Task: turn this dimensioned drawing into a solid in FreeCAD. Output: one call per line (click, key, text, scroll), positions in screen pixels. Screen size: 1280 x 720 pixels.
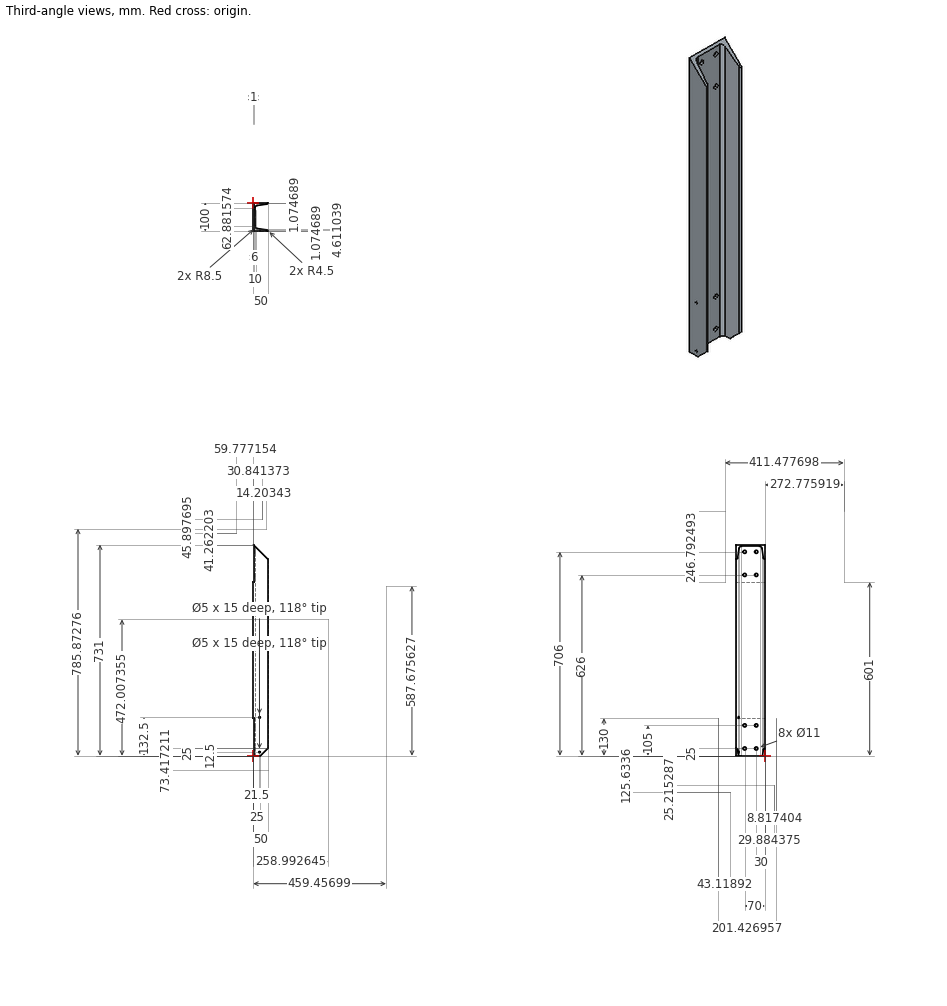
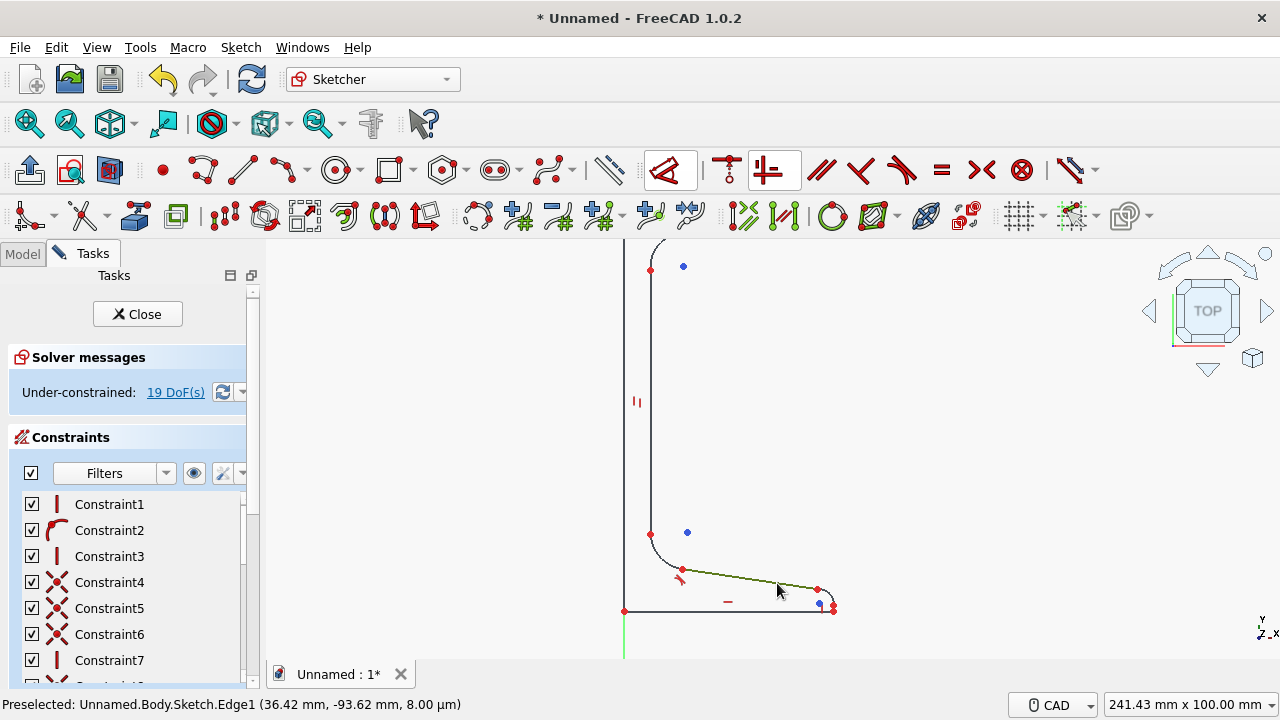
click(830, 594)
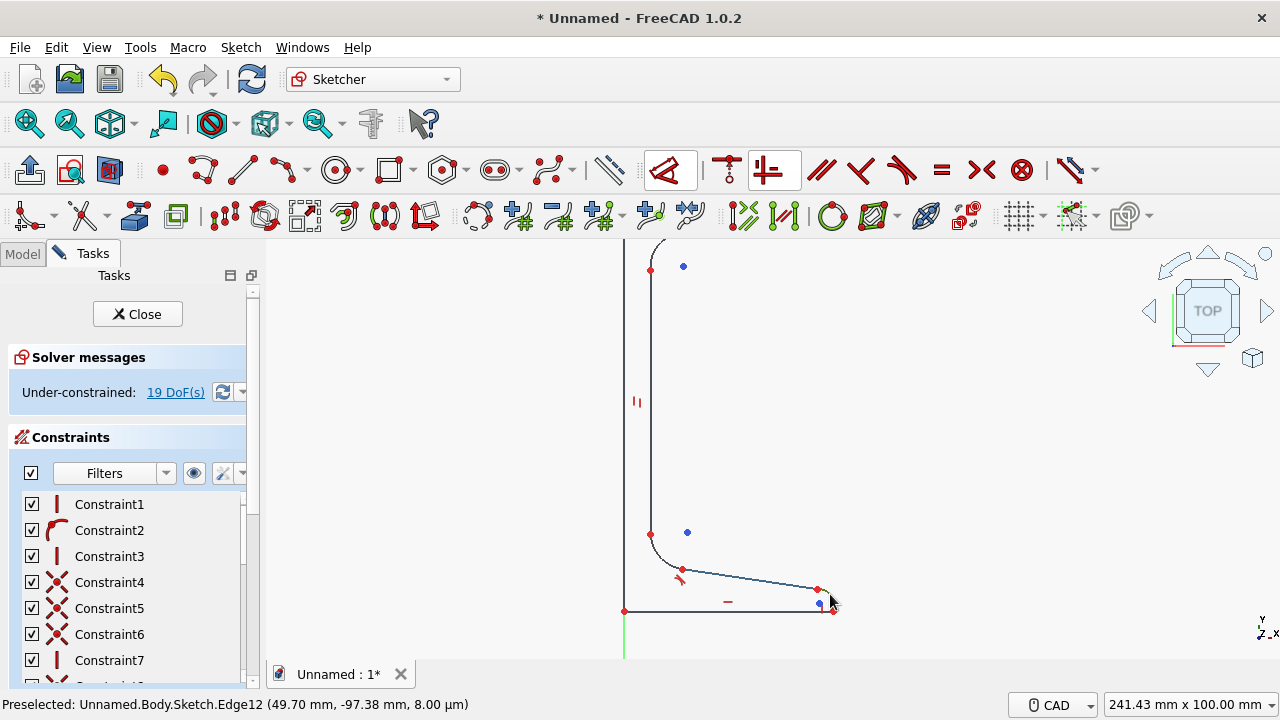
key(t)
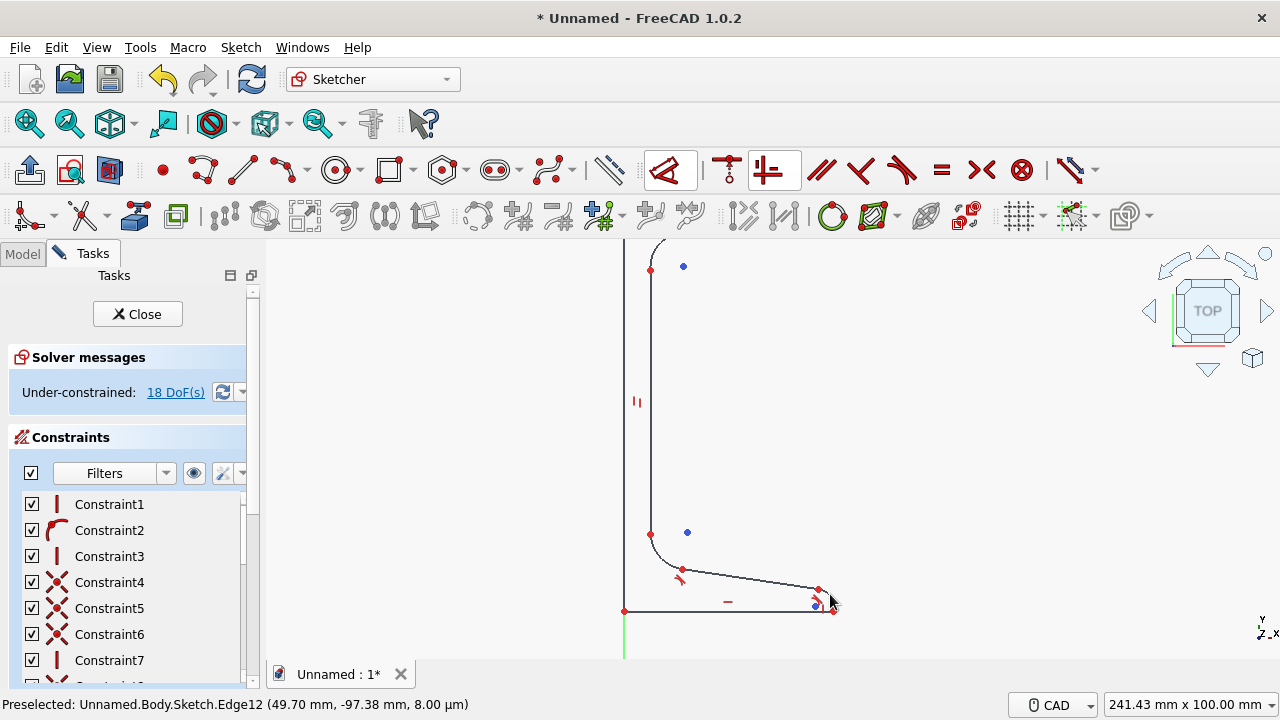
click(651, 455)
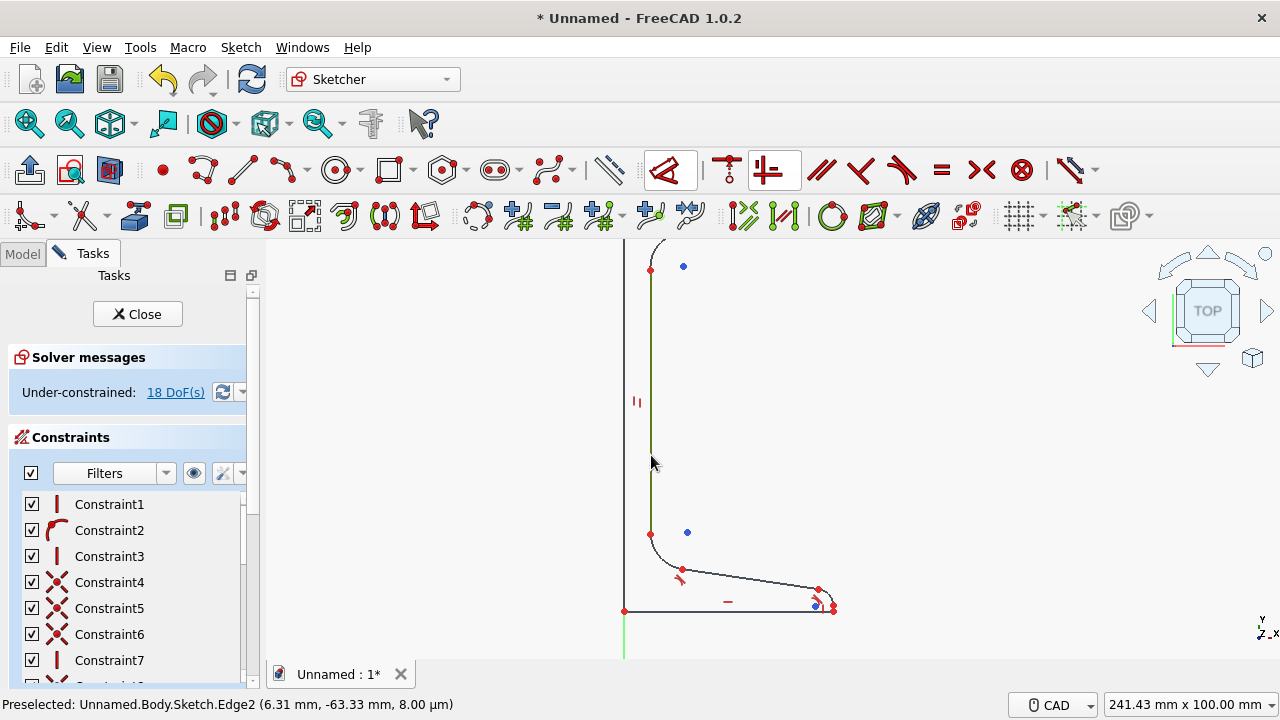
click(655, 549)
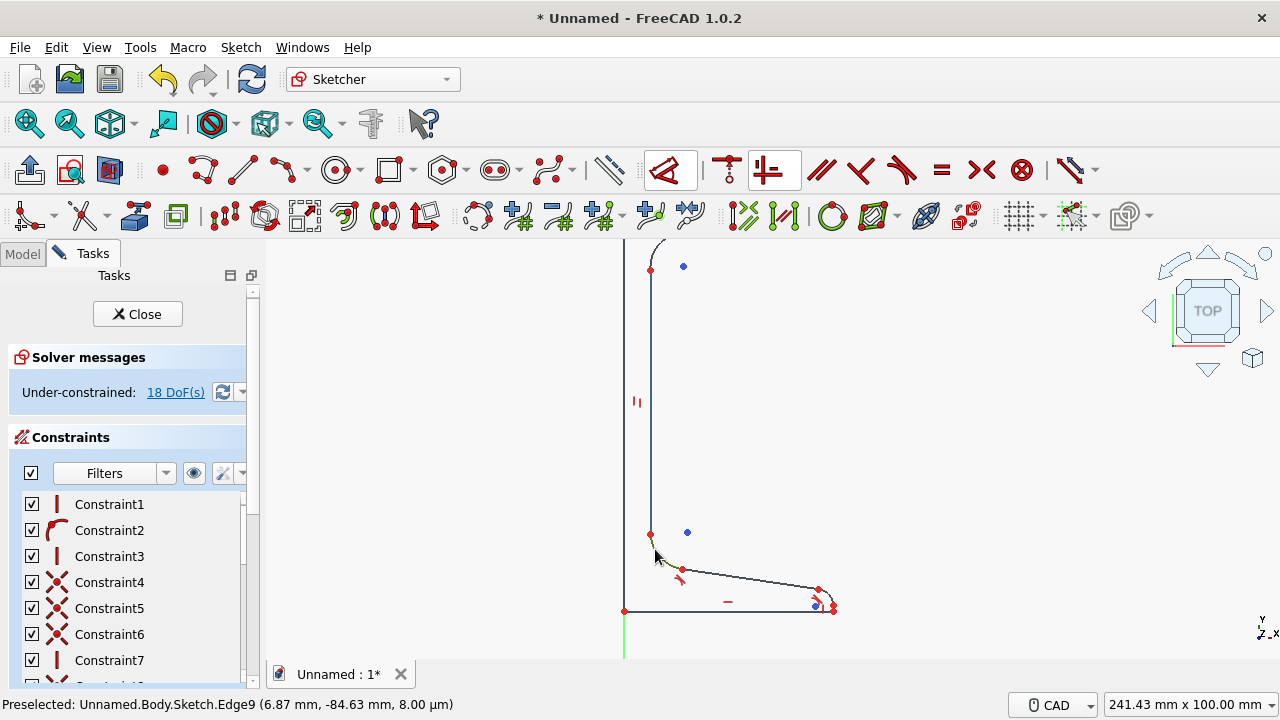
key(t)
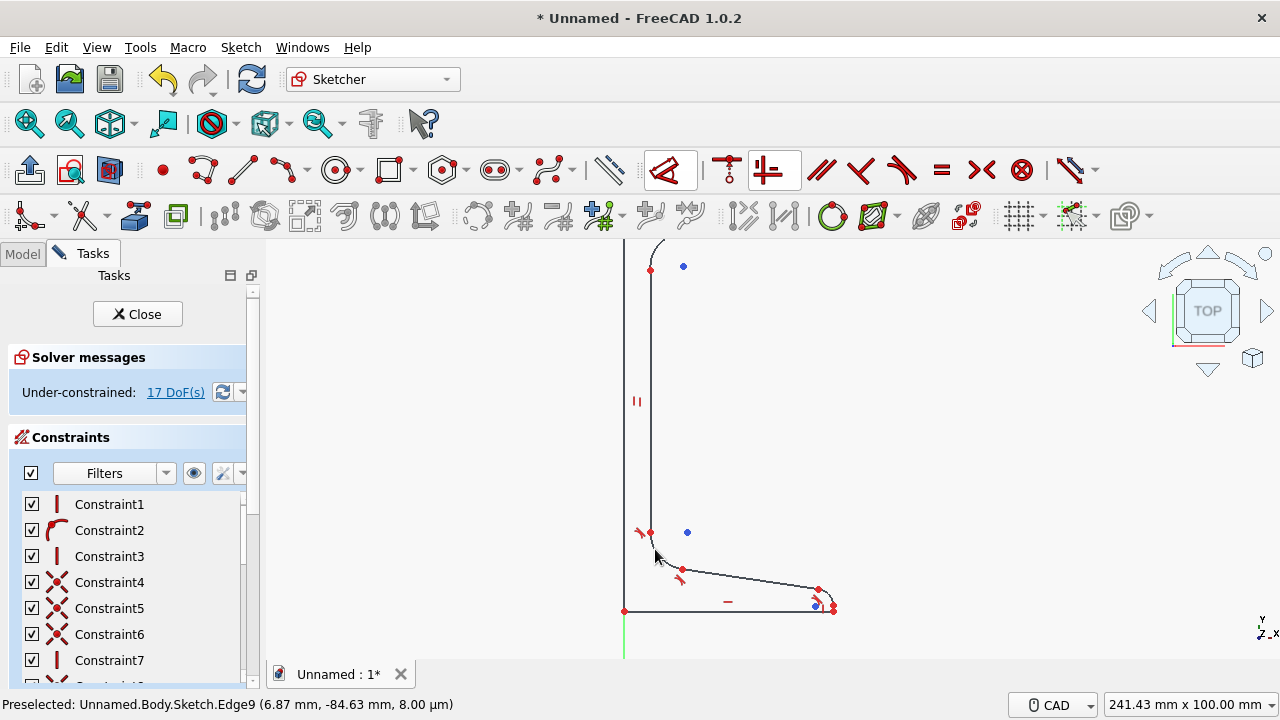
click(651, 454)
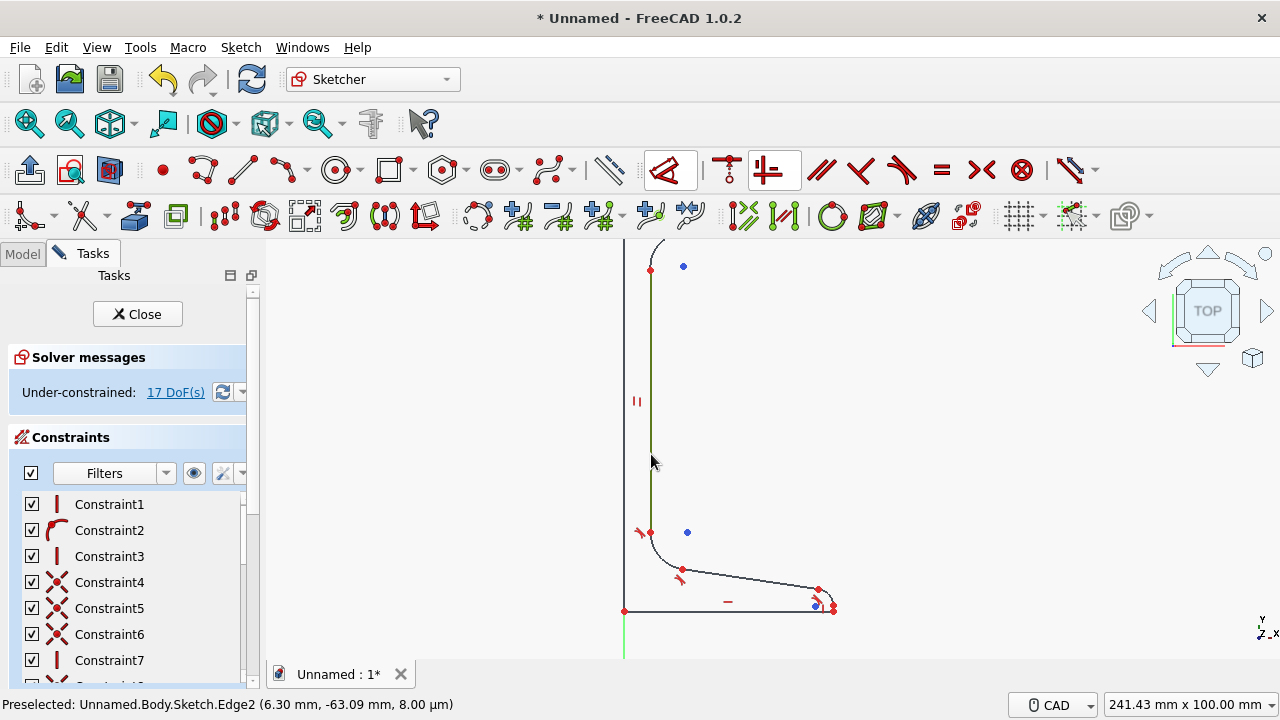
scroll(654, 549, down, 2)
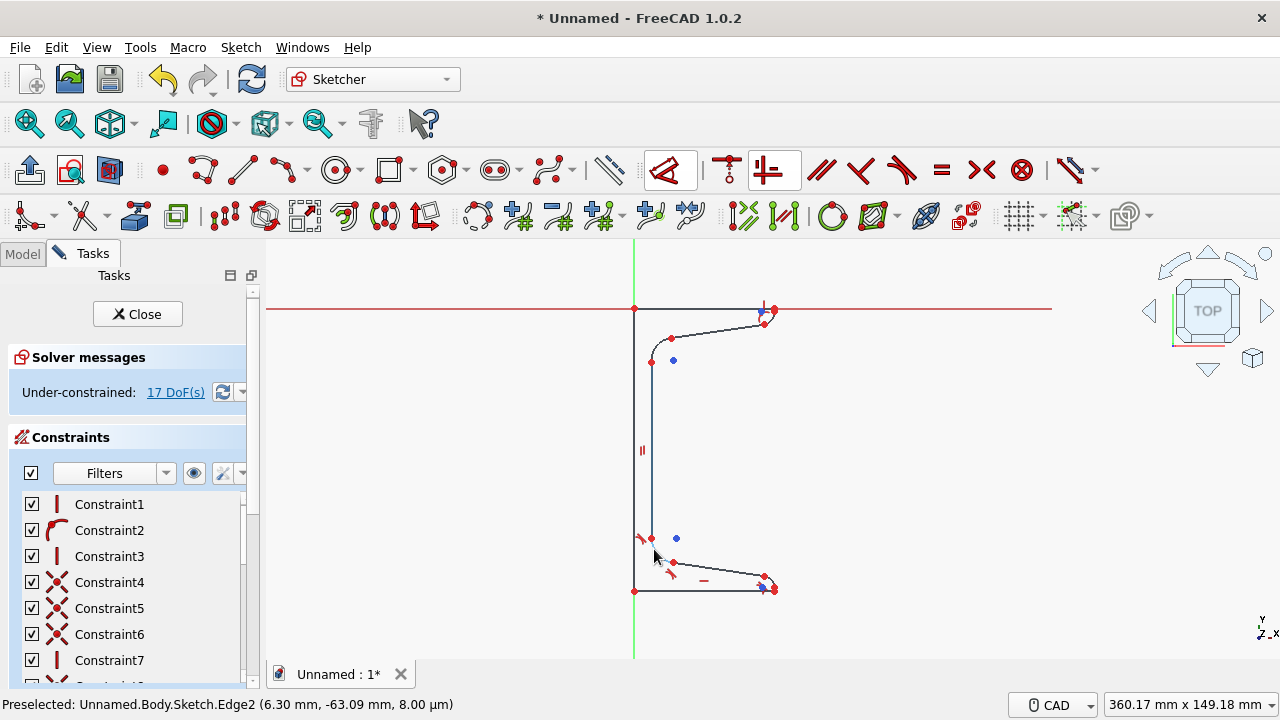
scroll(662, 342, up, 2)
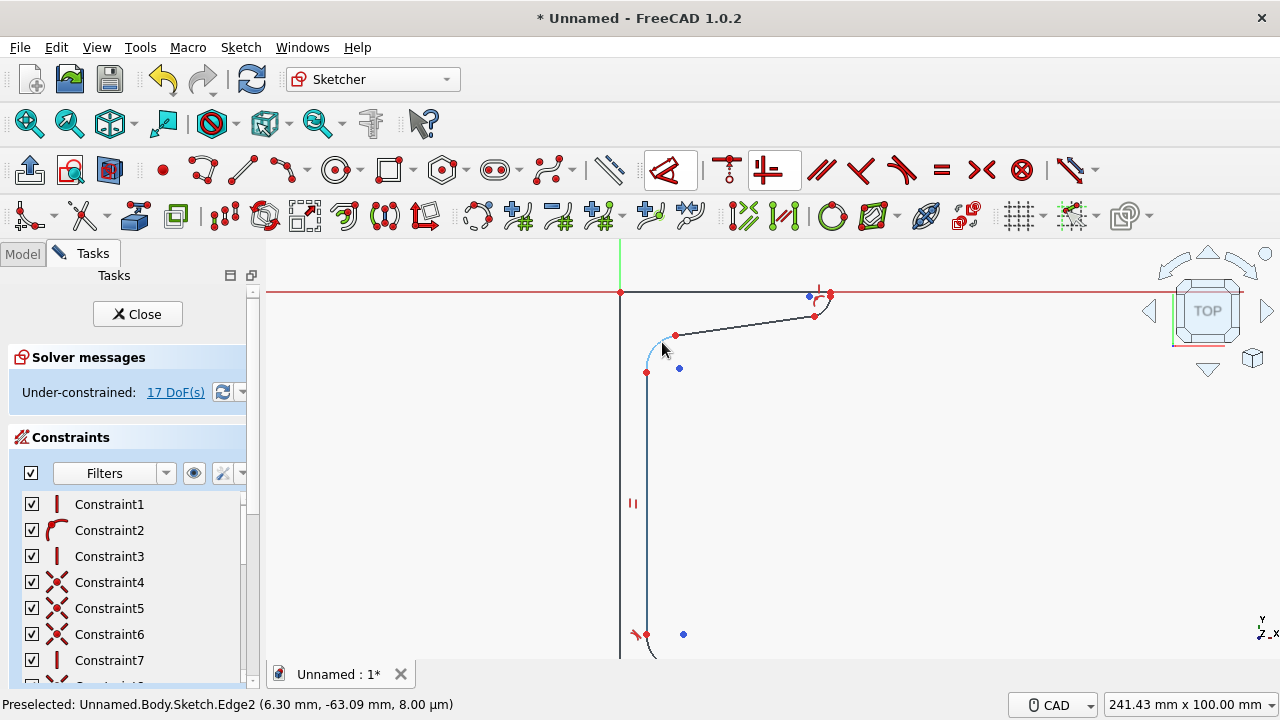
click(661, 341)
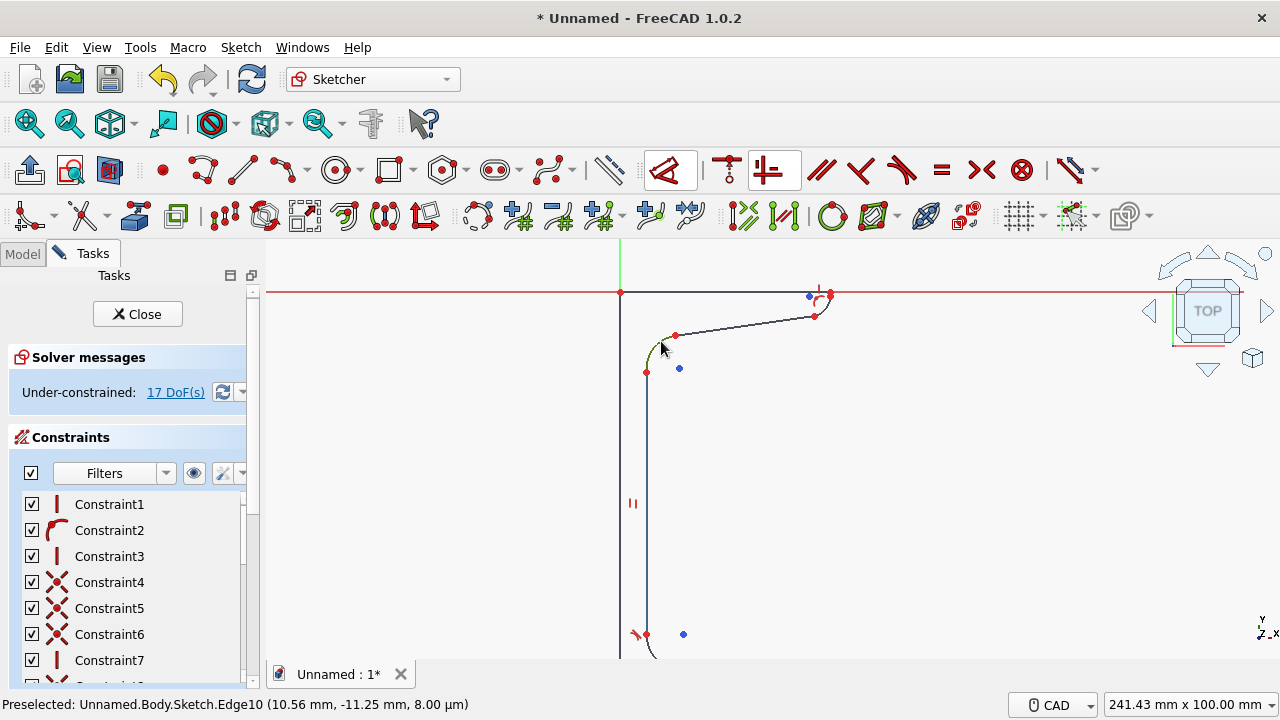
click(902, 170)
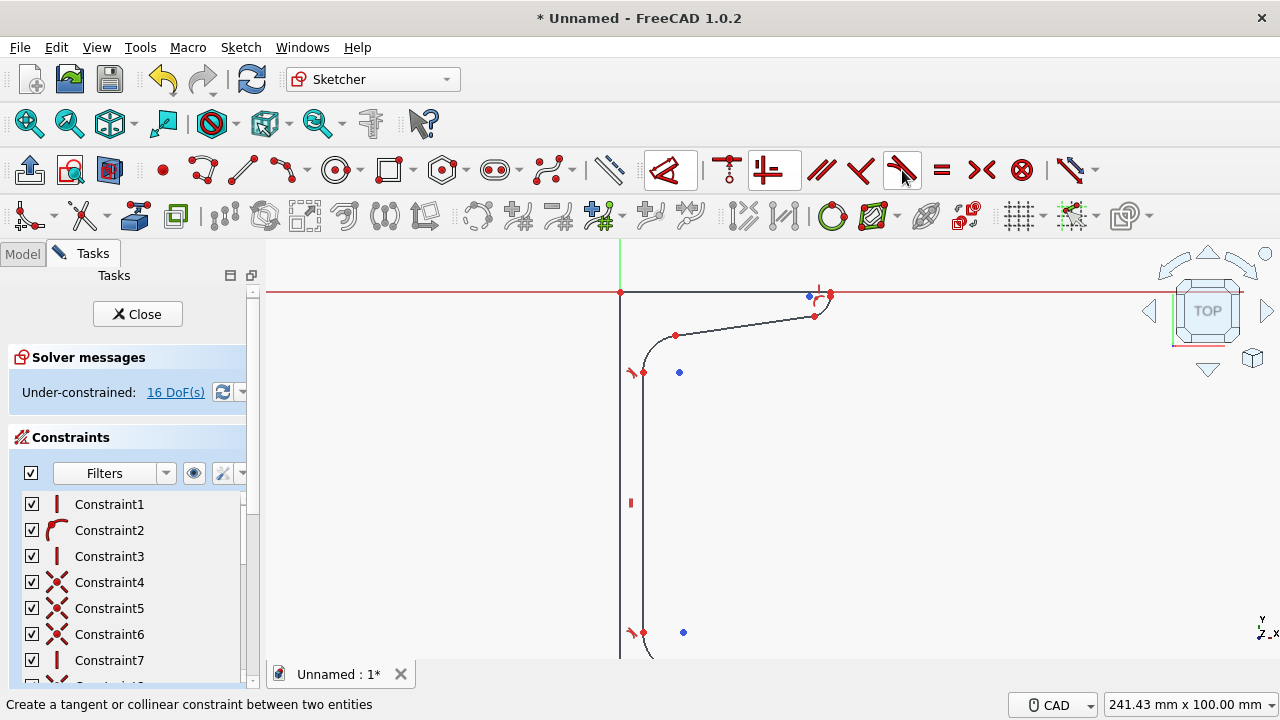
click(717, 330)